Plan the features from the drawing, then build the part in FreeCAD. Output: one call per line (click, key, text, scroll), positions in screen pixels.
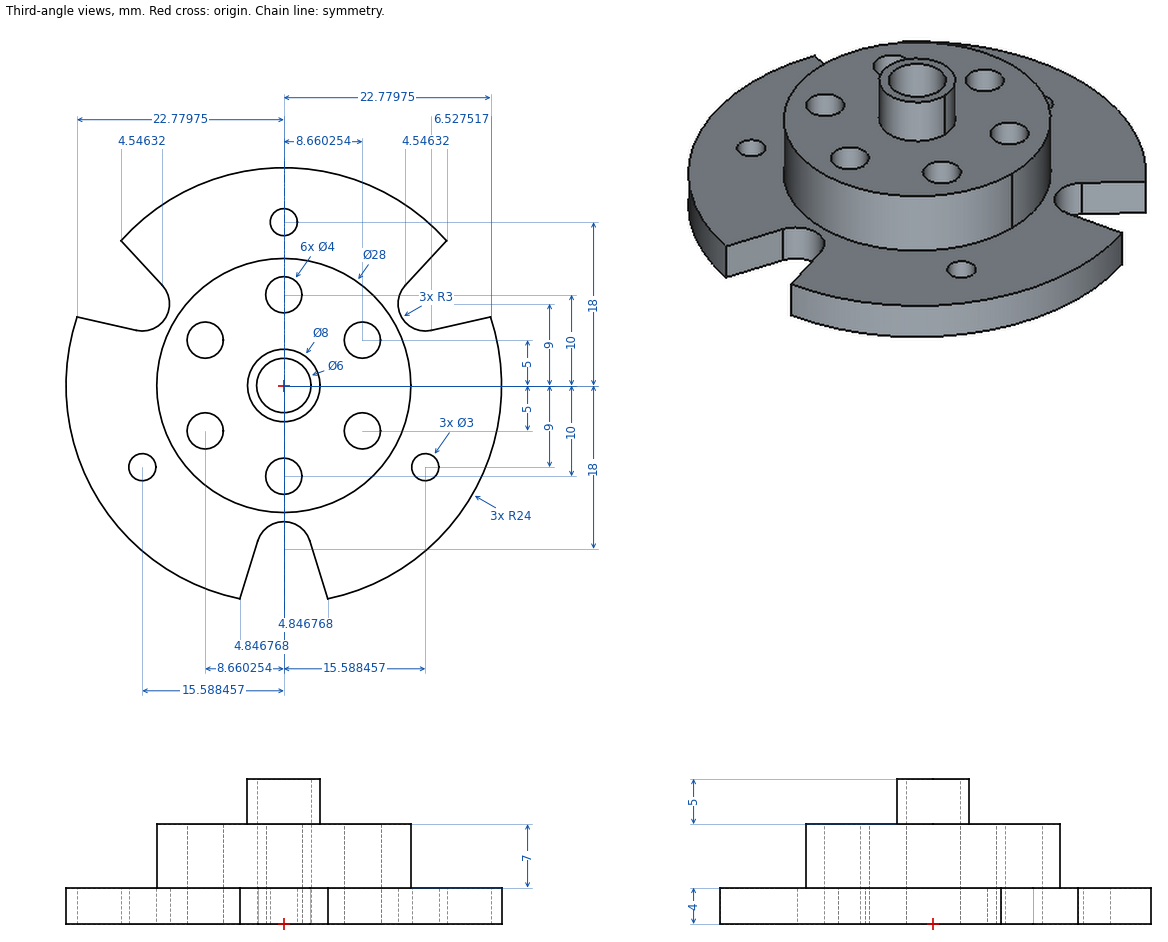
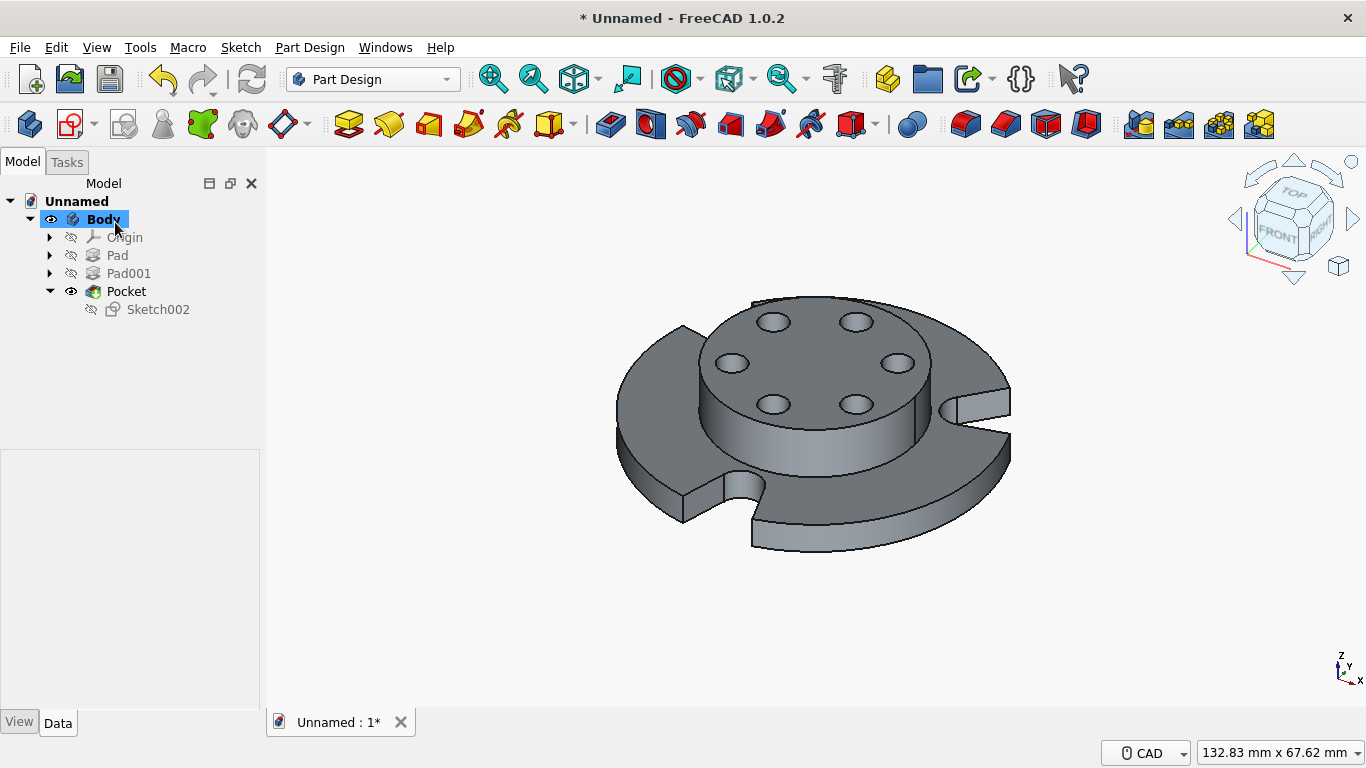
click(815, 362)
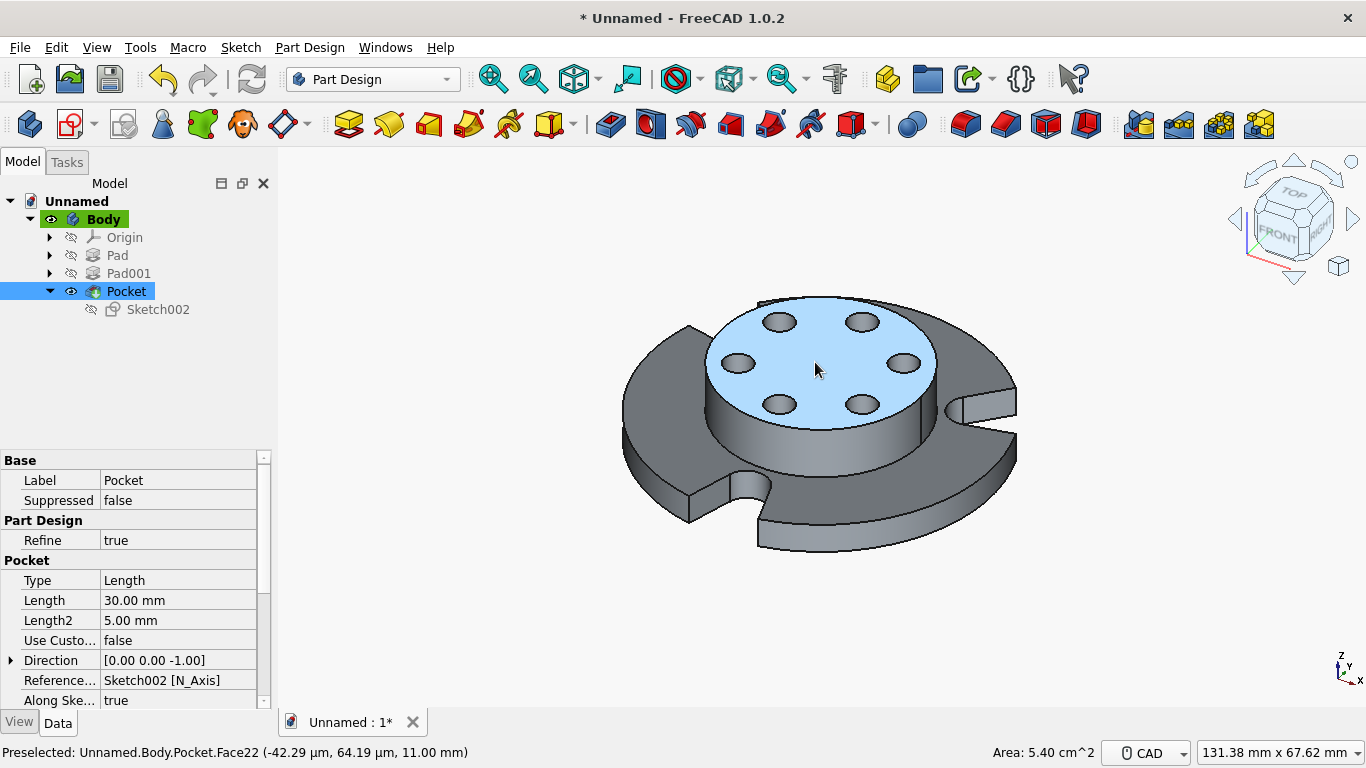
click(70, 124)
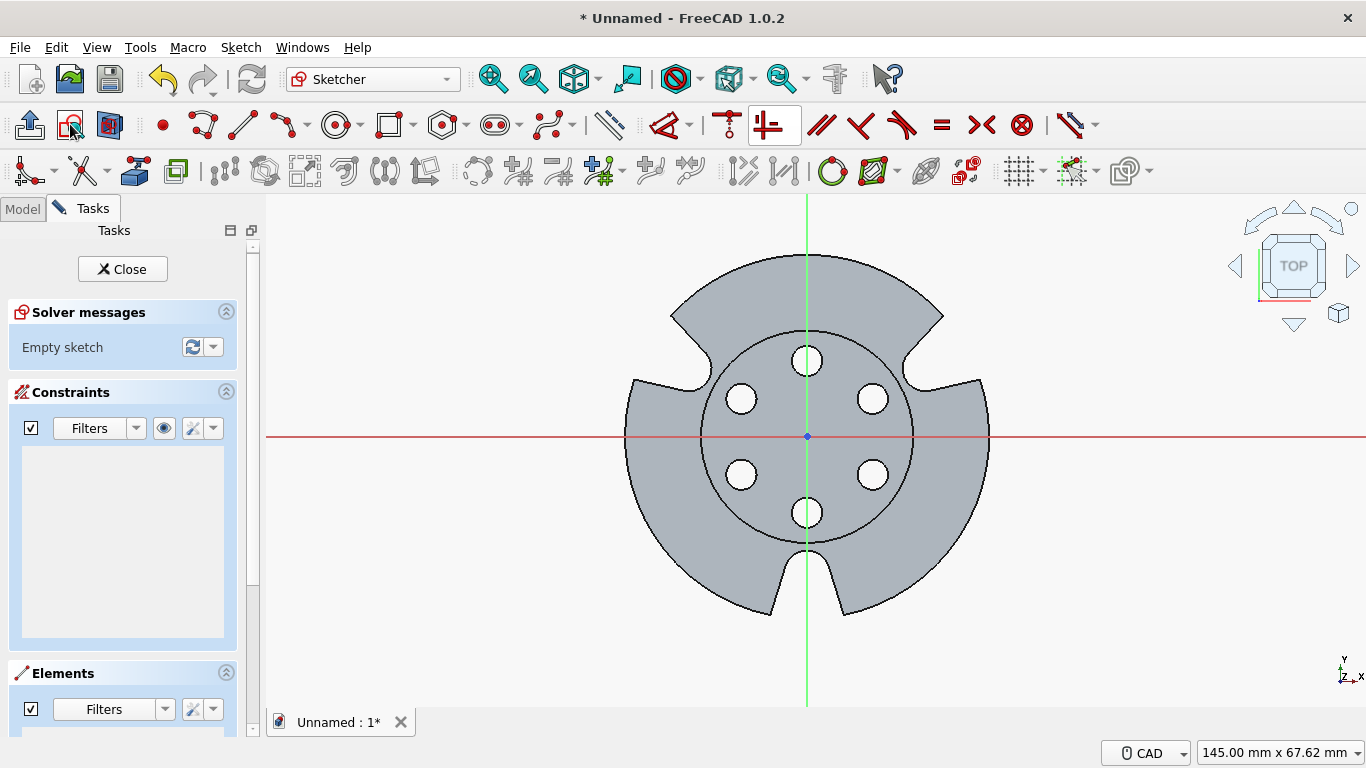
scroll(822, 433, up, 8)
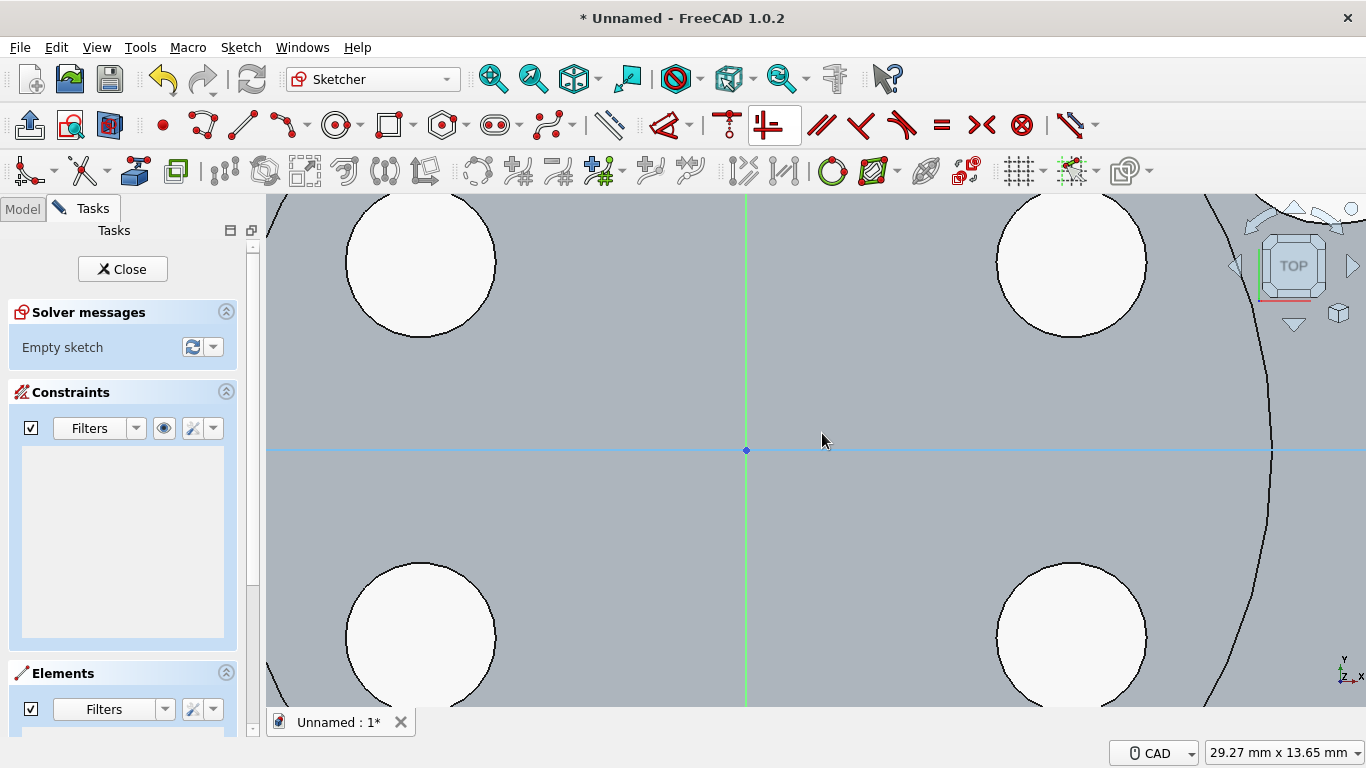
key(g)
key(c)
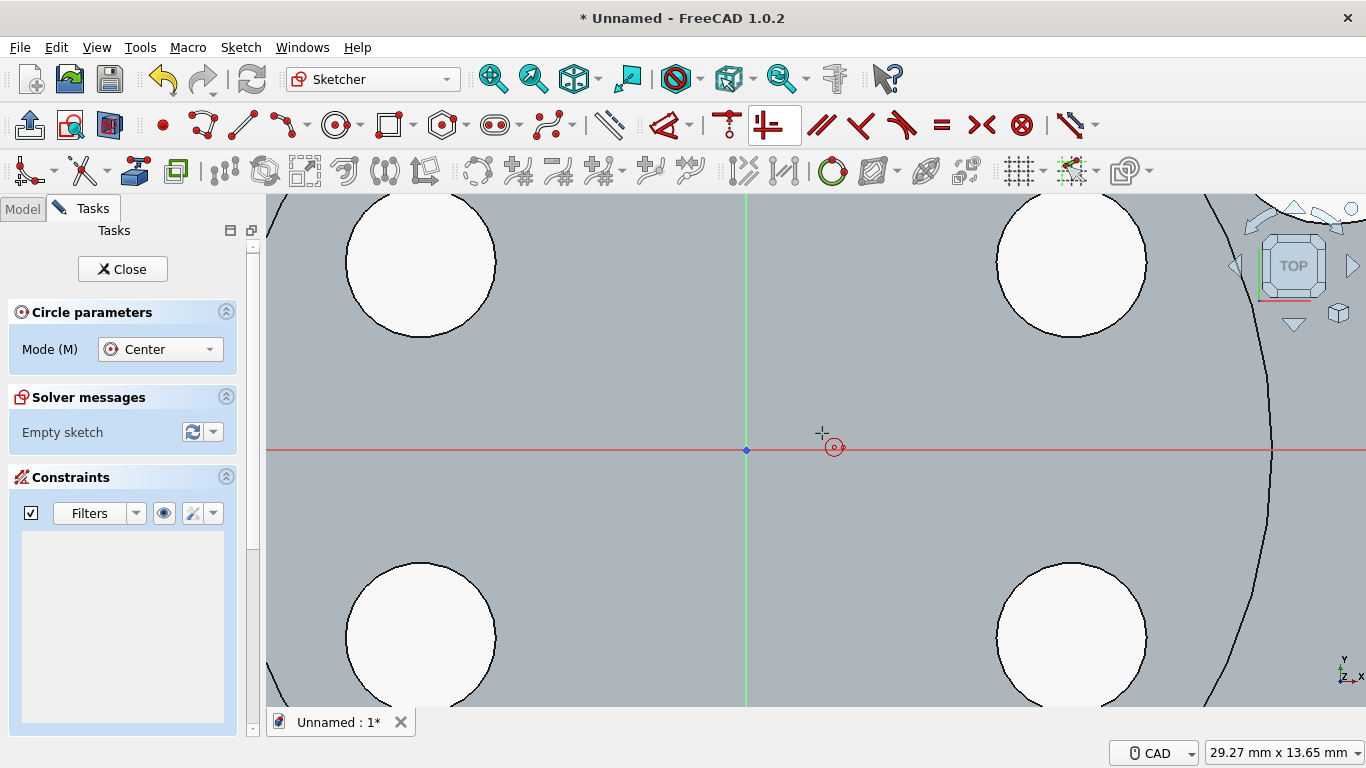
click(746, 450)
click(852, 344)
key(Escape)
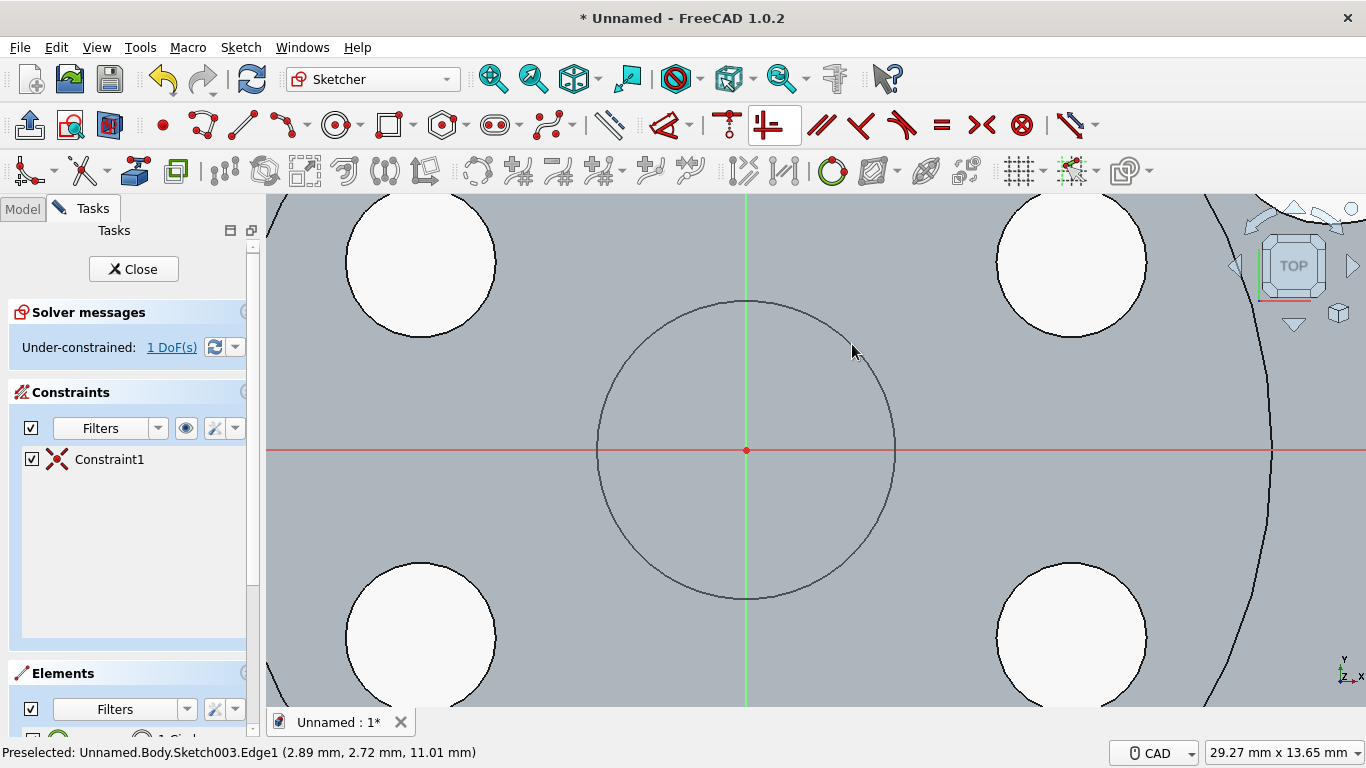
click(664, 126)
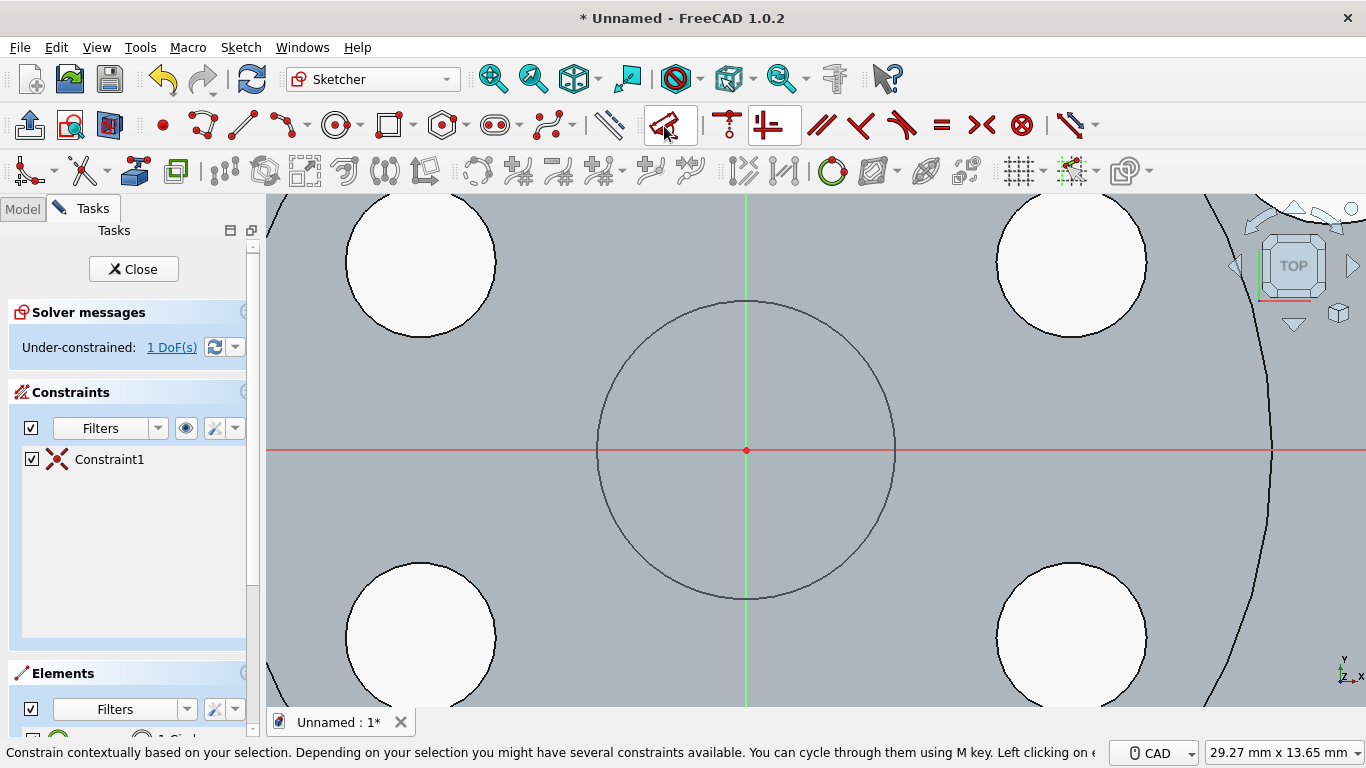
click(851, 344)
click(873, 321)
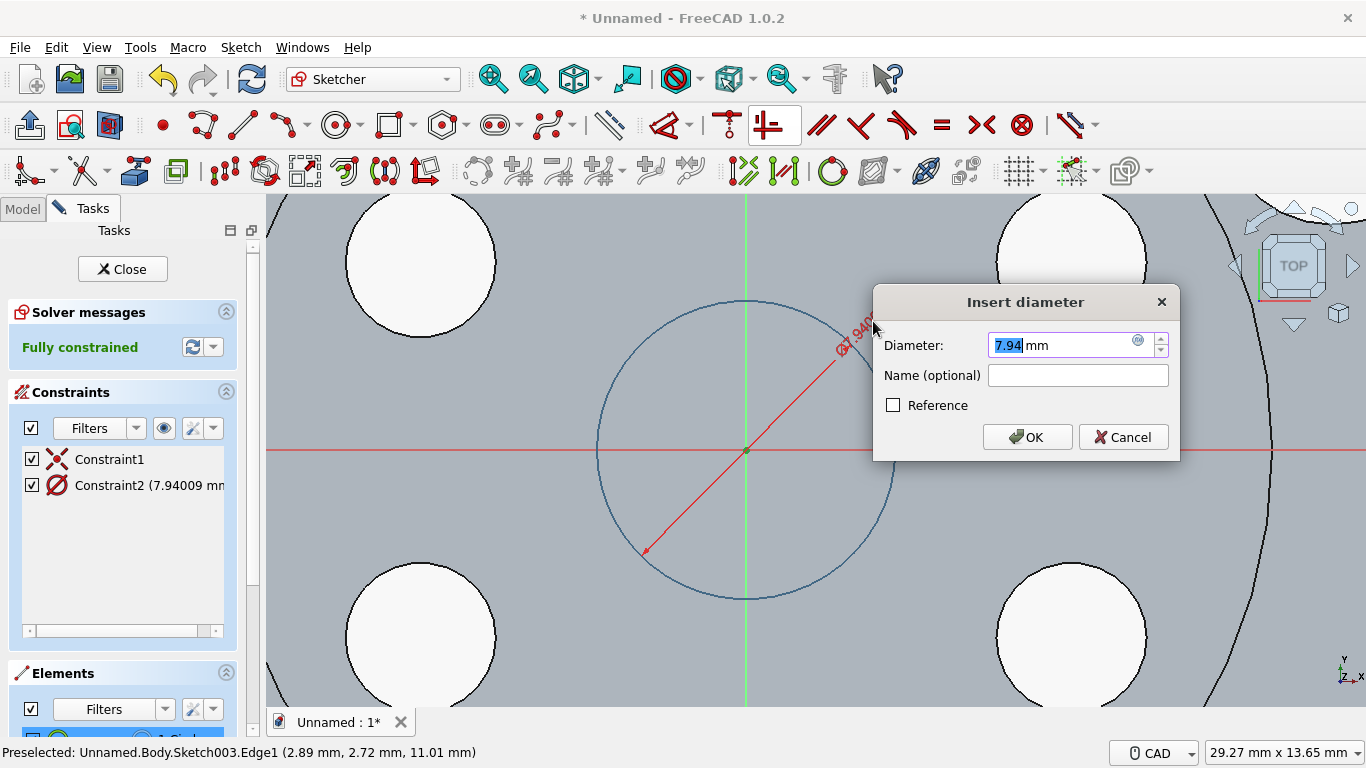
text(8)
key(Return)
key(Escape)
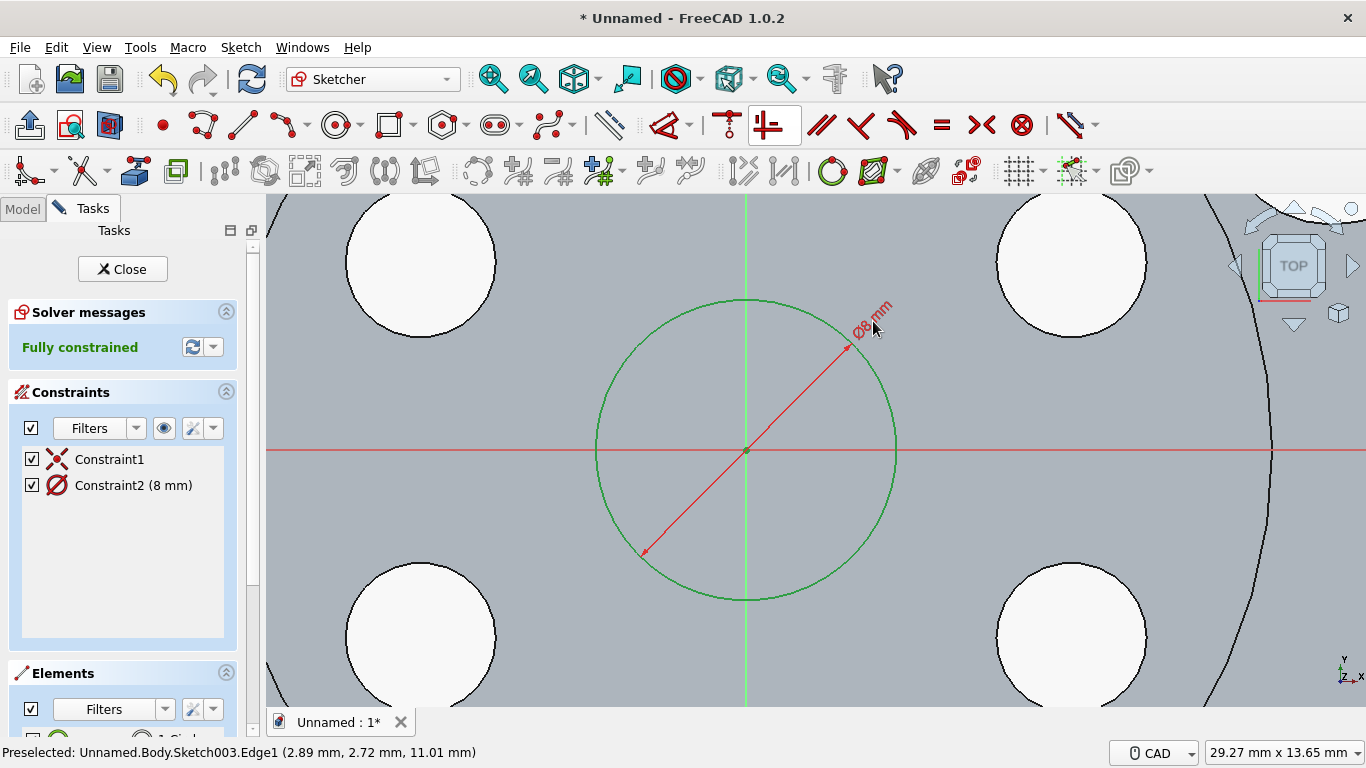
click(123, 269)